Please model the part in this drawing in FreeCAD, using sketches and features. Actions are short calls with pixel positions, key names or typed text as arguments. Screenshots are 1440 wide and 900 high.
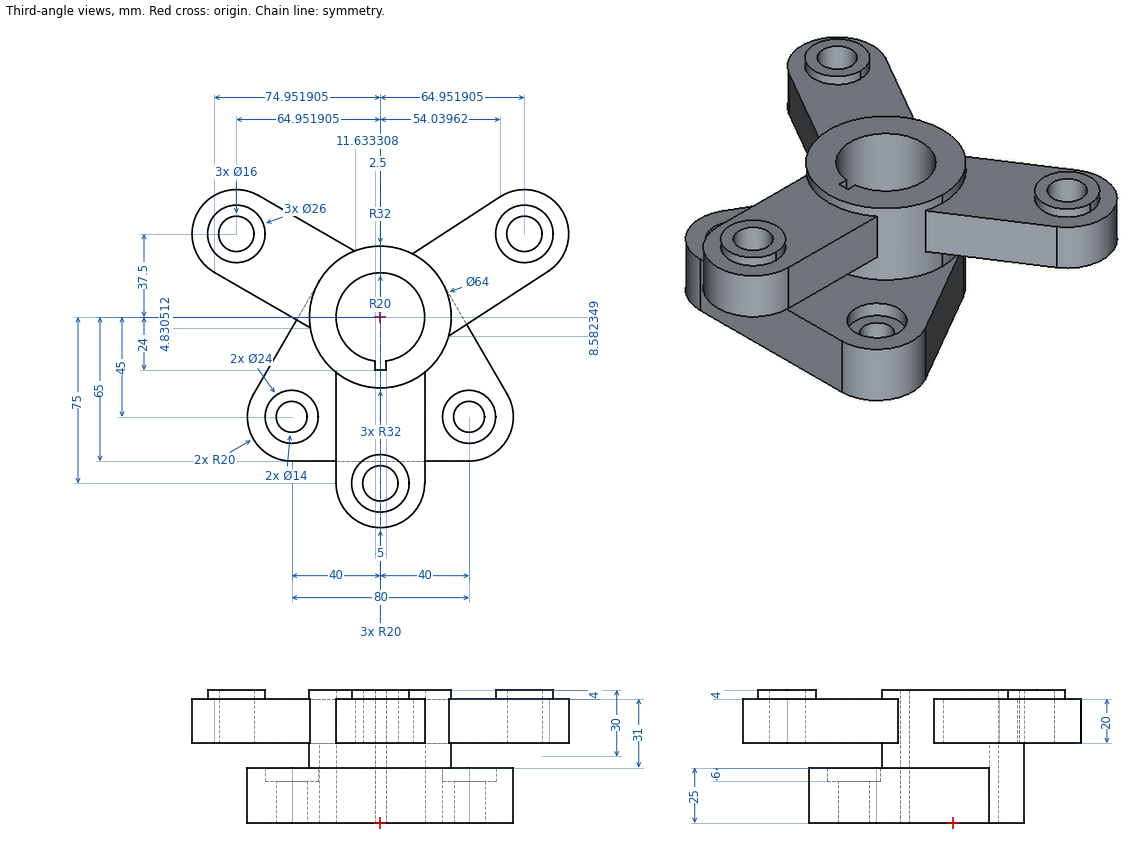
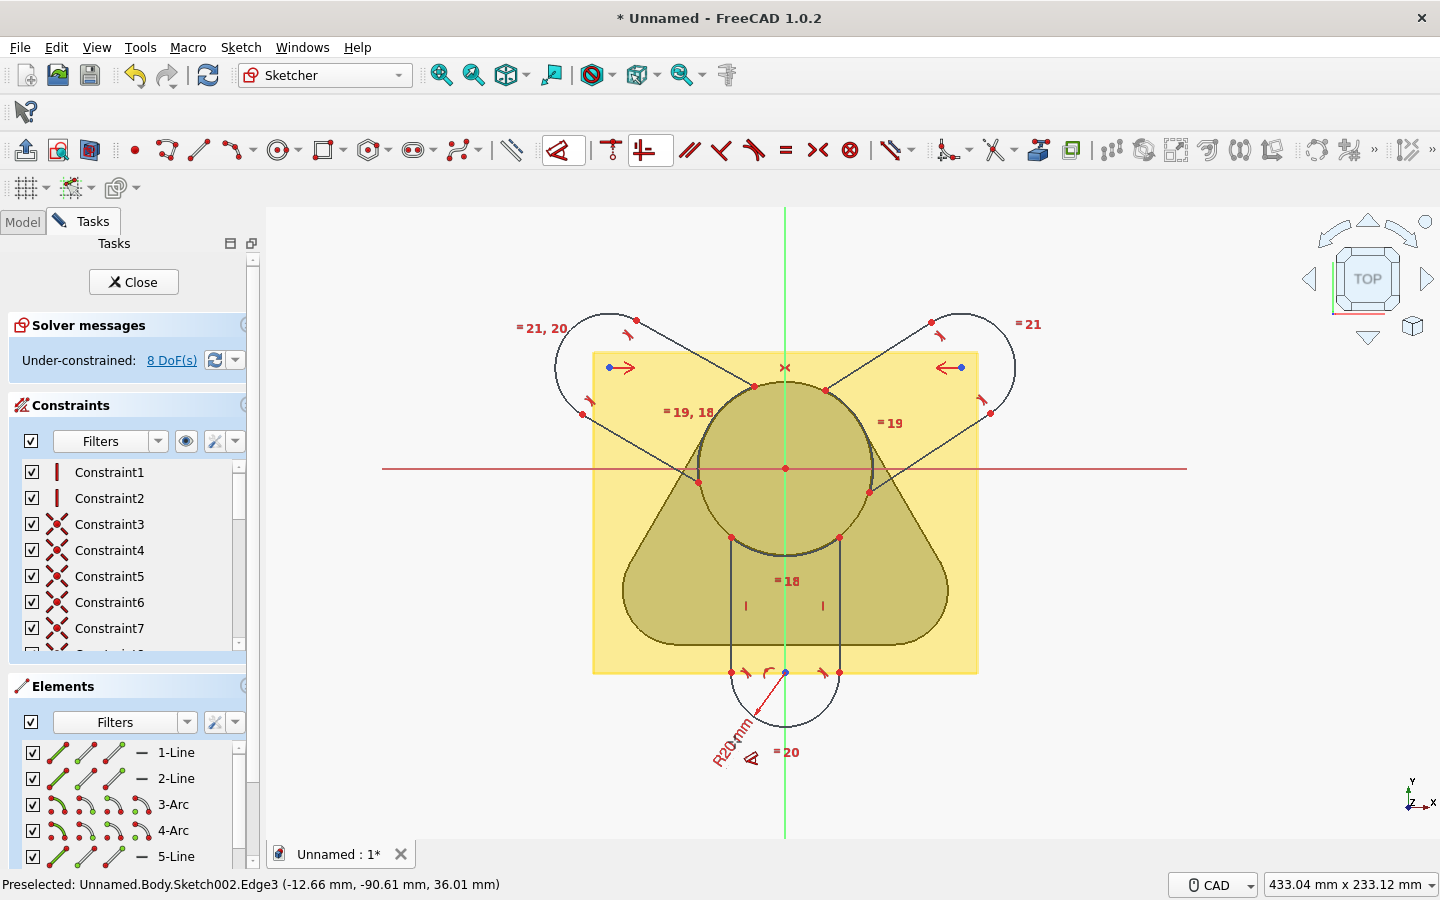
click(762, 553)
click(753, 584)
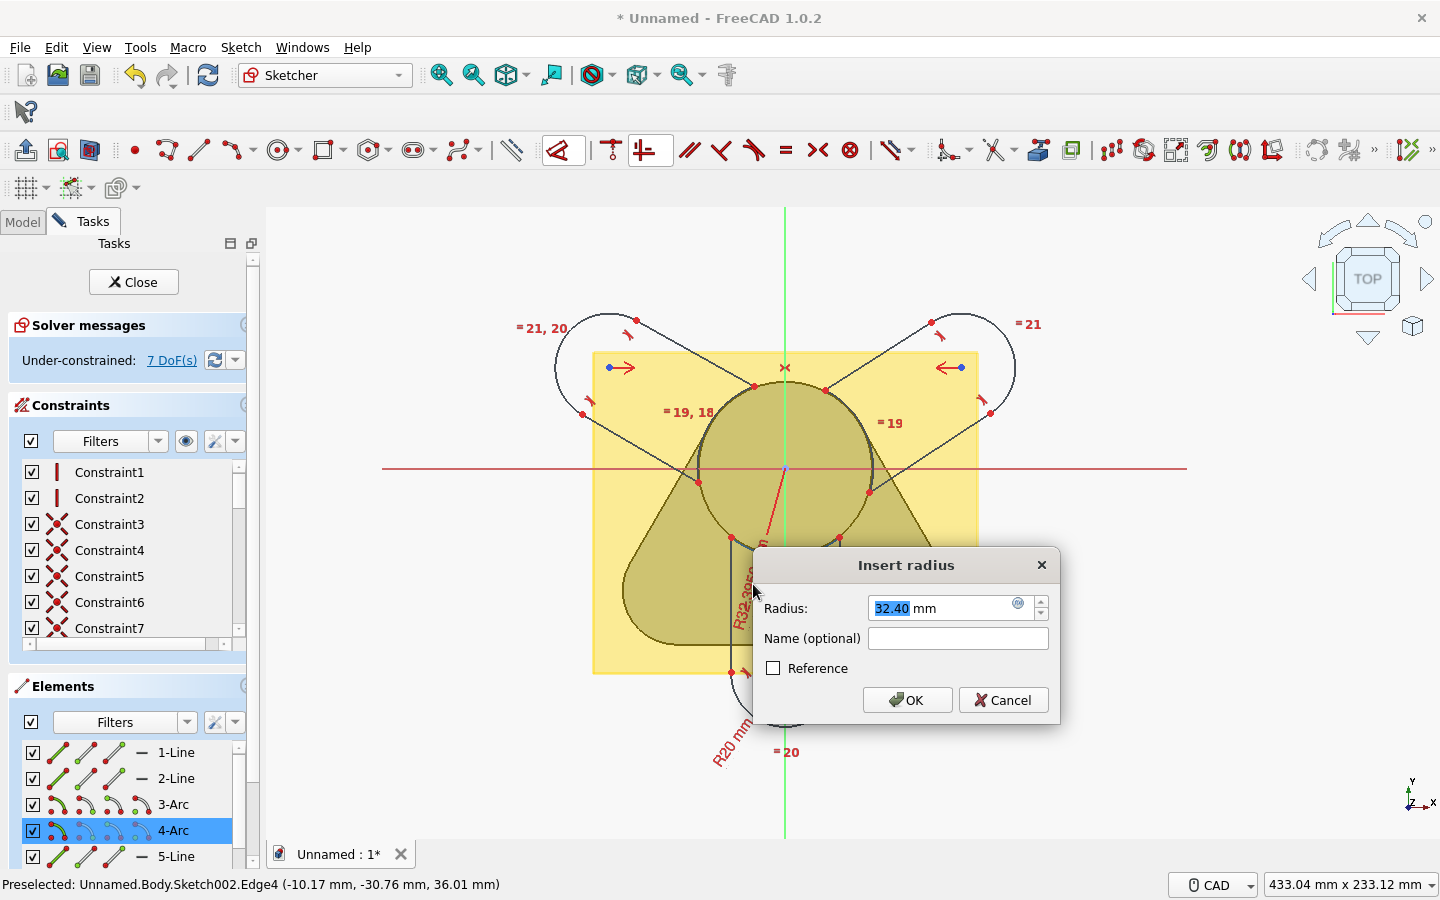
text(32)
key(Return)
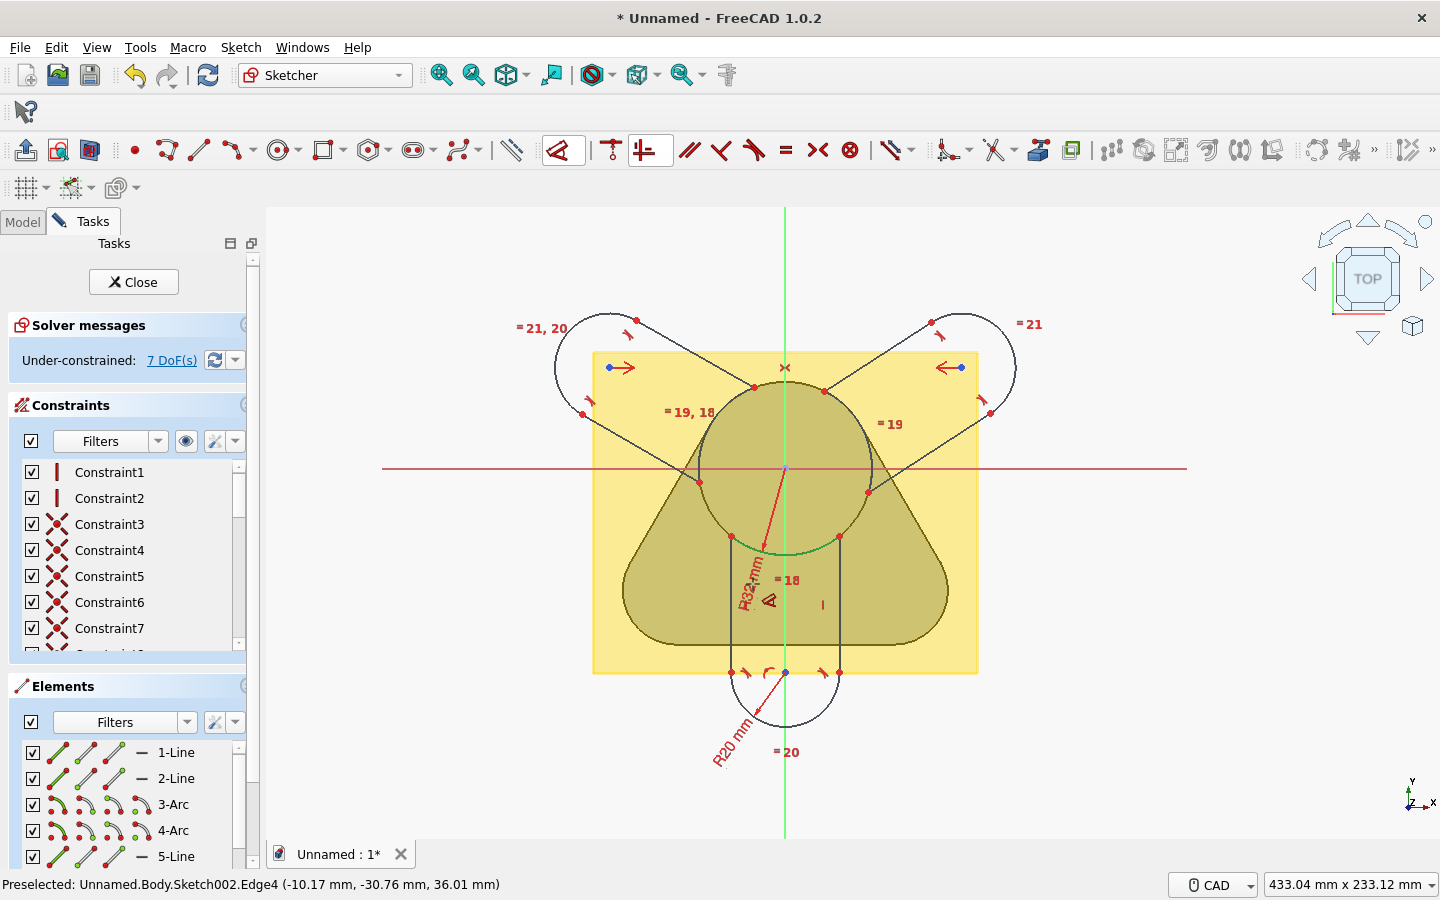
click(731, 673)
click(697, 524)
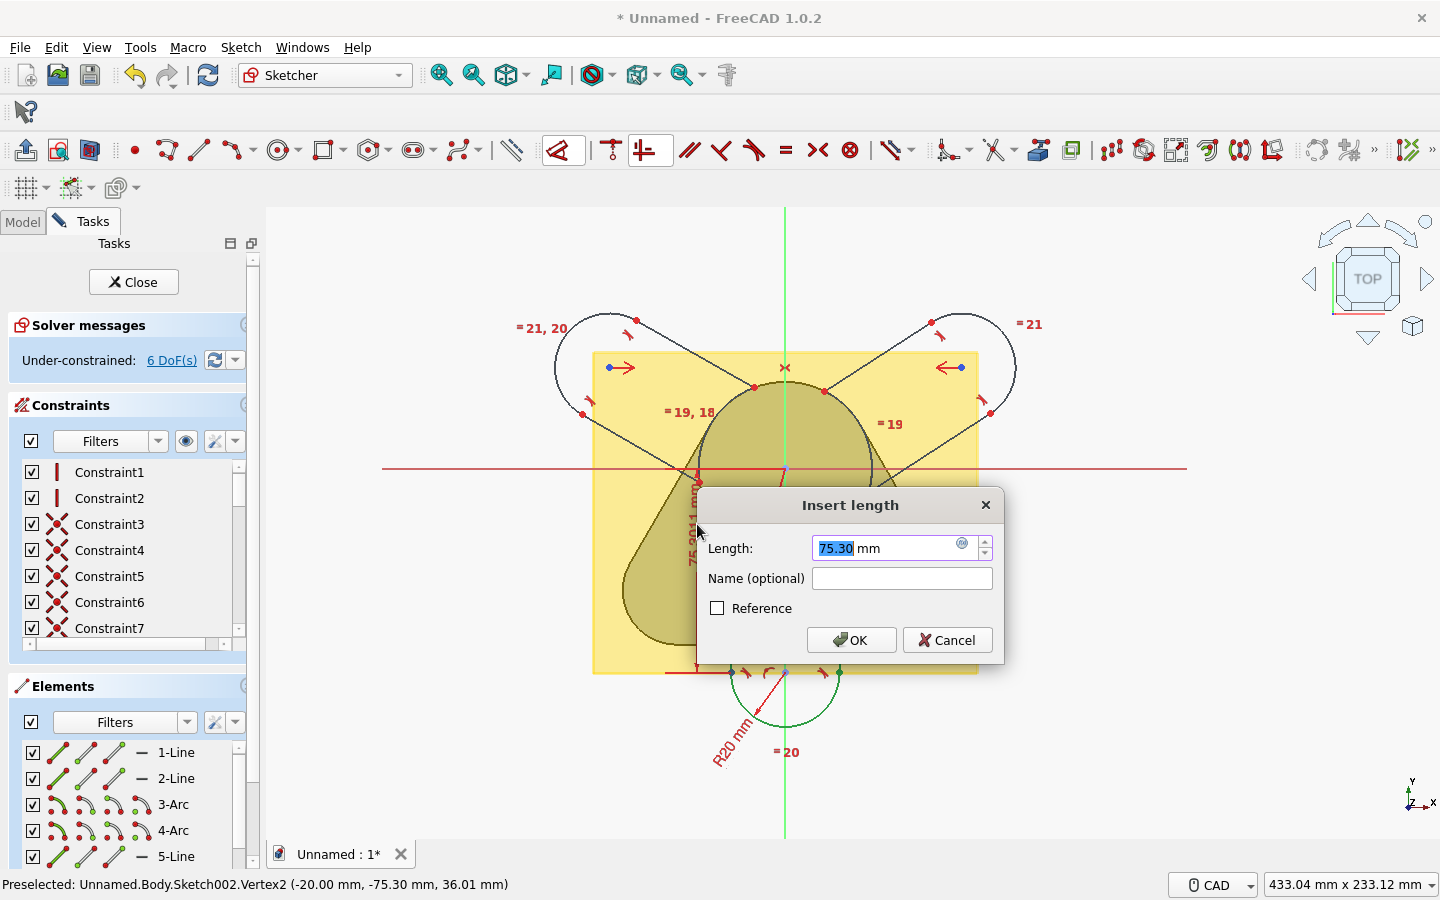
text(75)
key(Return)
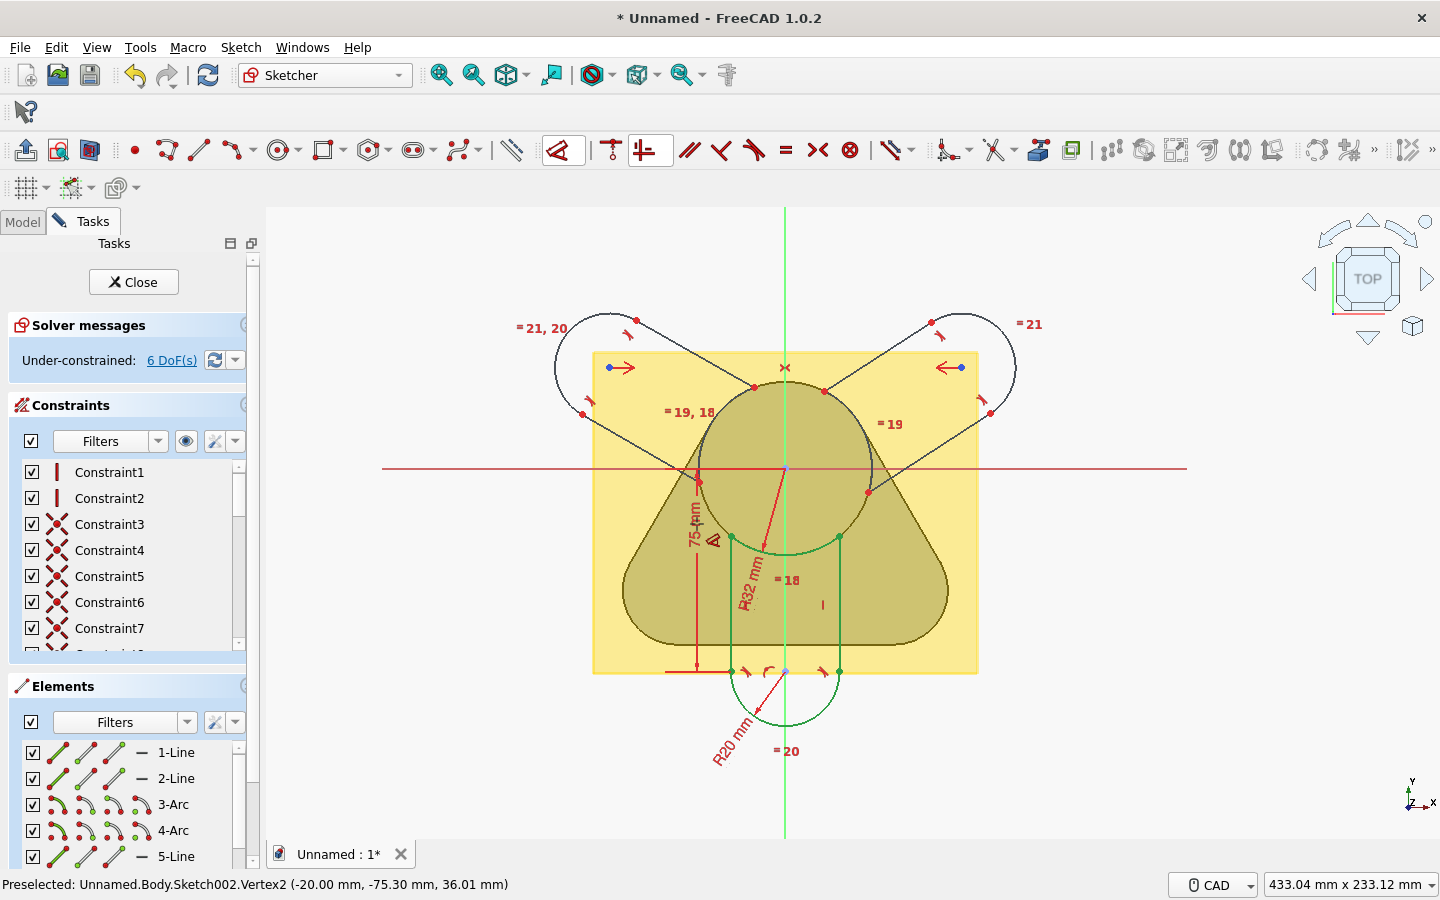
click(609, 368)
click(575, 441)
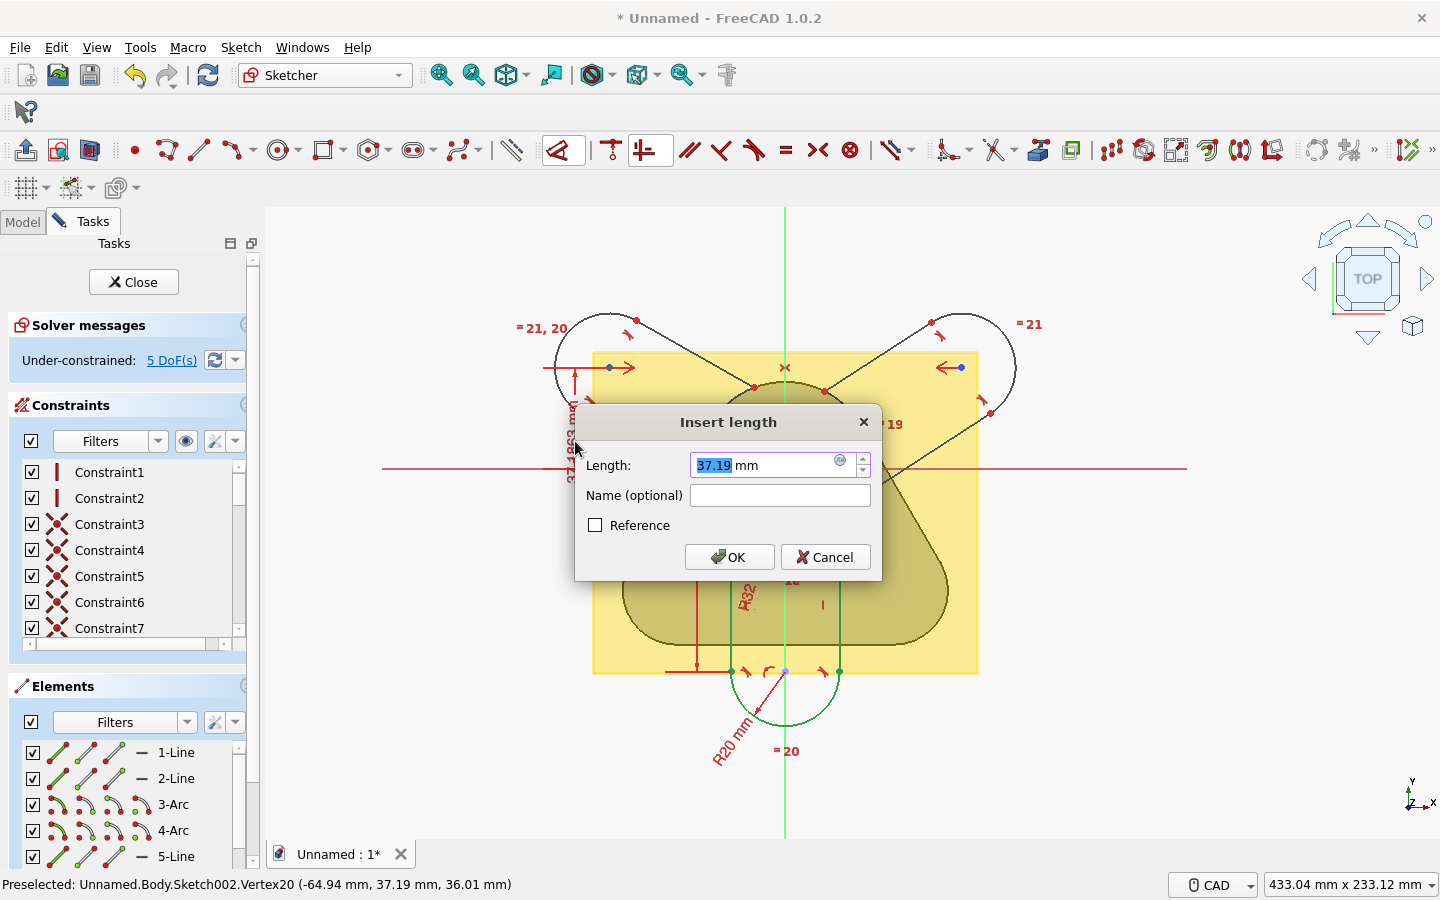
text(37.5)
key(Return)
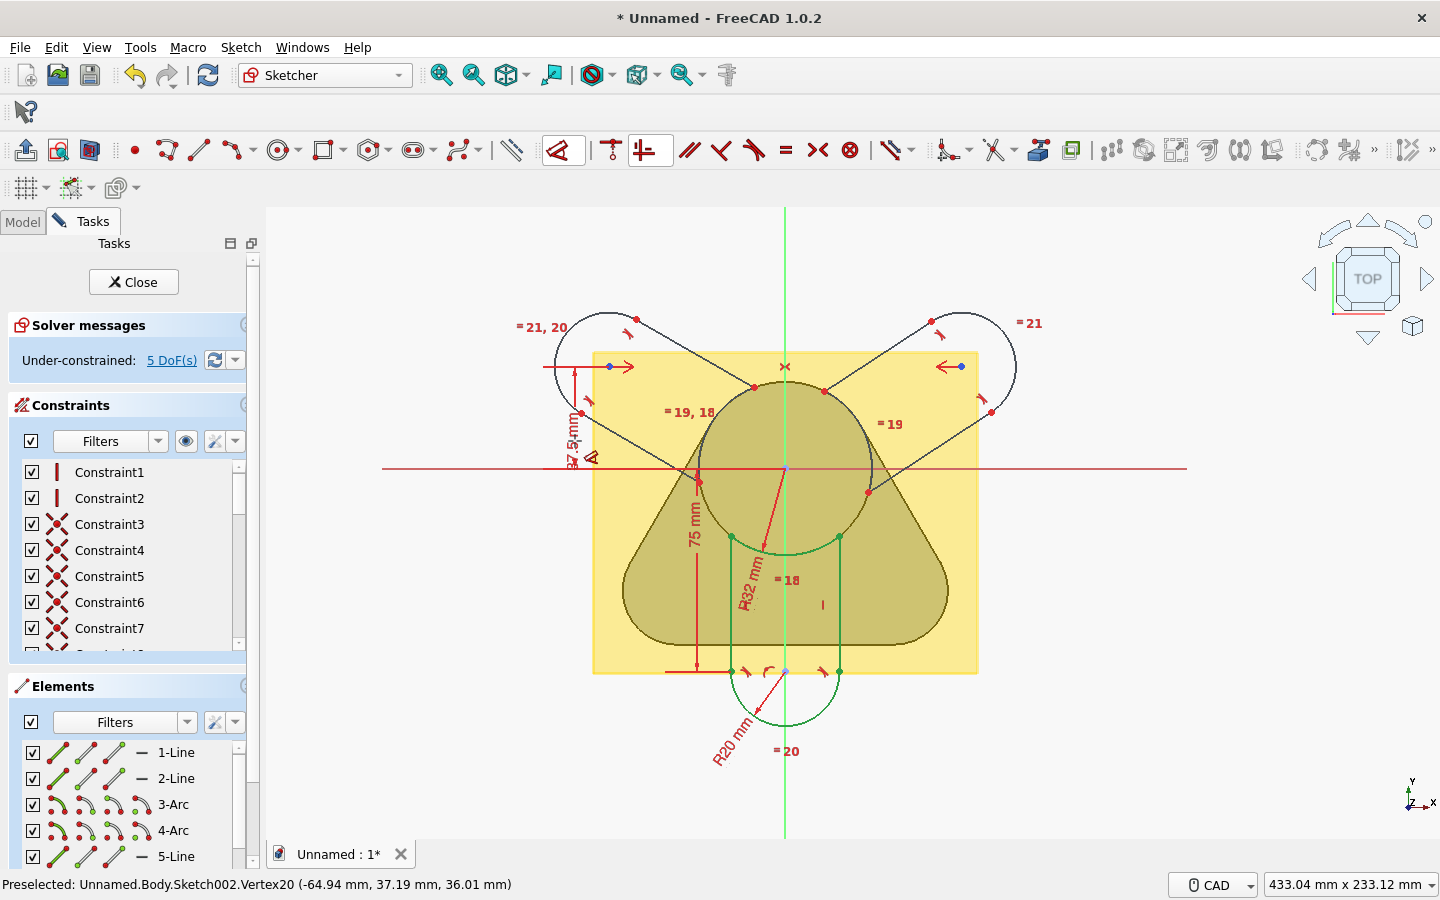
scroll(700, 483, up, 6)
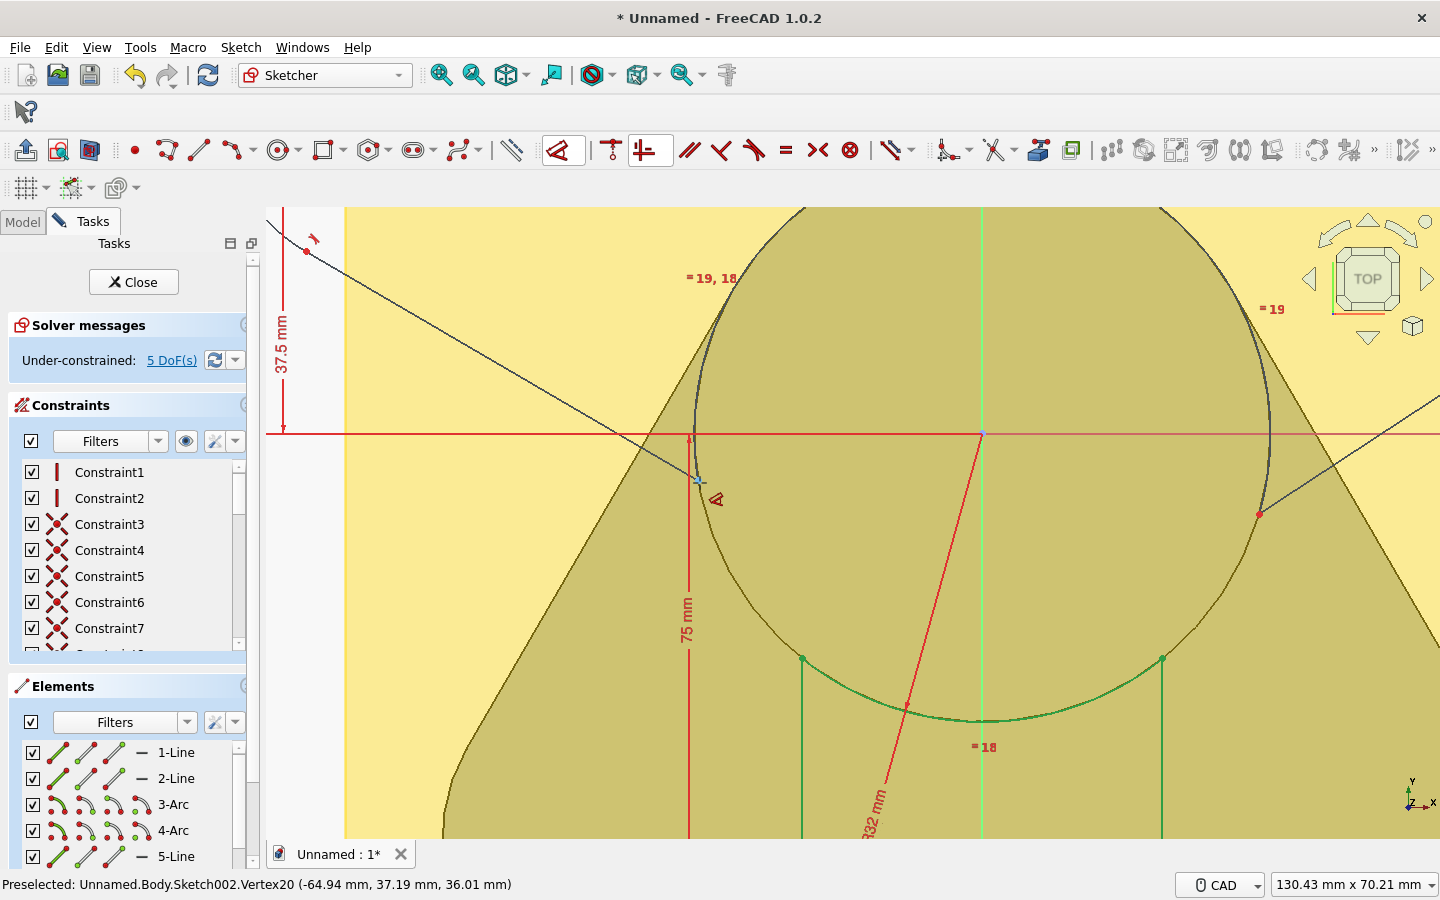
click(698, 481)
click(1016, 457)